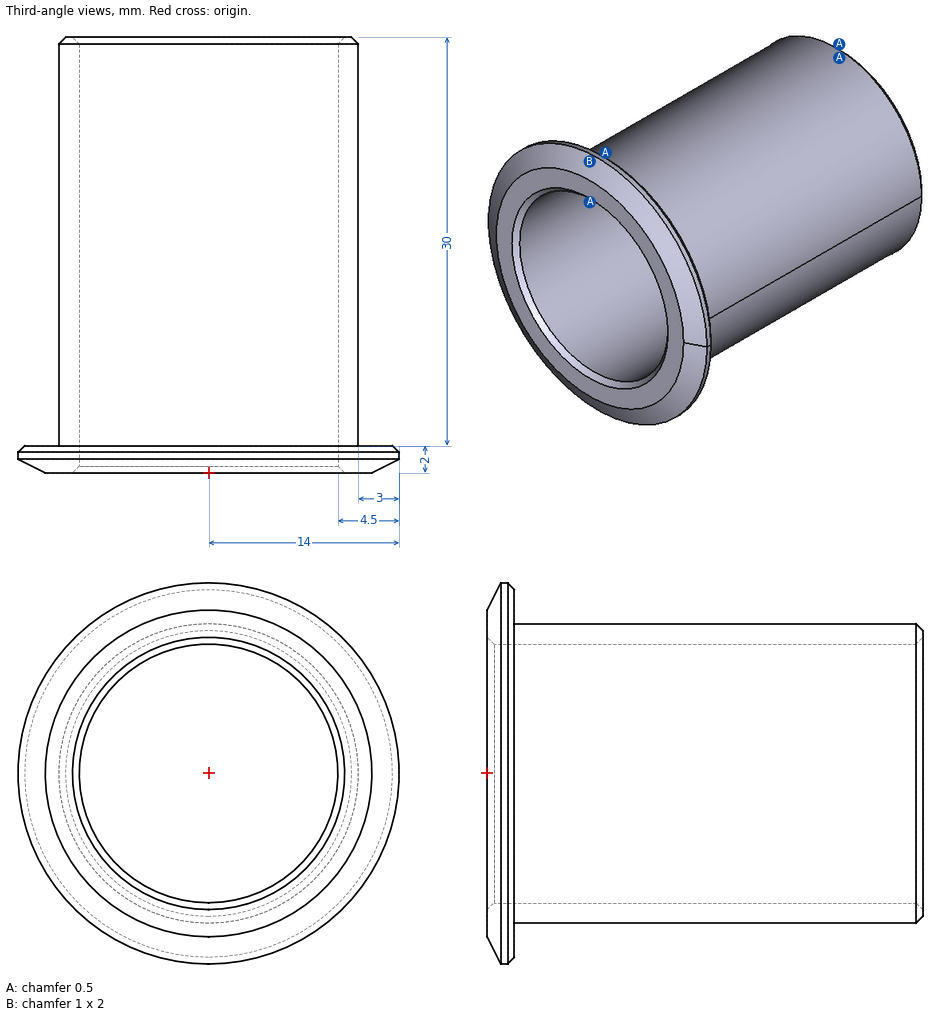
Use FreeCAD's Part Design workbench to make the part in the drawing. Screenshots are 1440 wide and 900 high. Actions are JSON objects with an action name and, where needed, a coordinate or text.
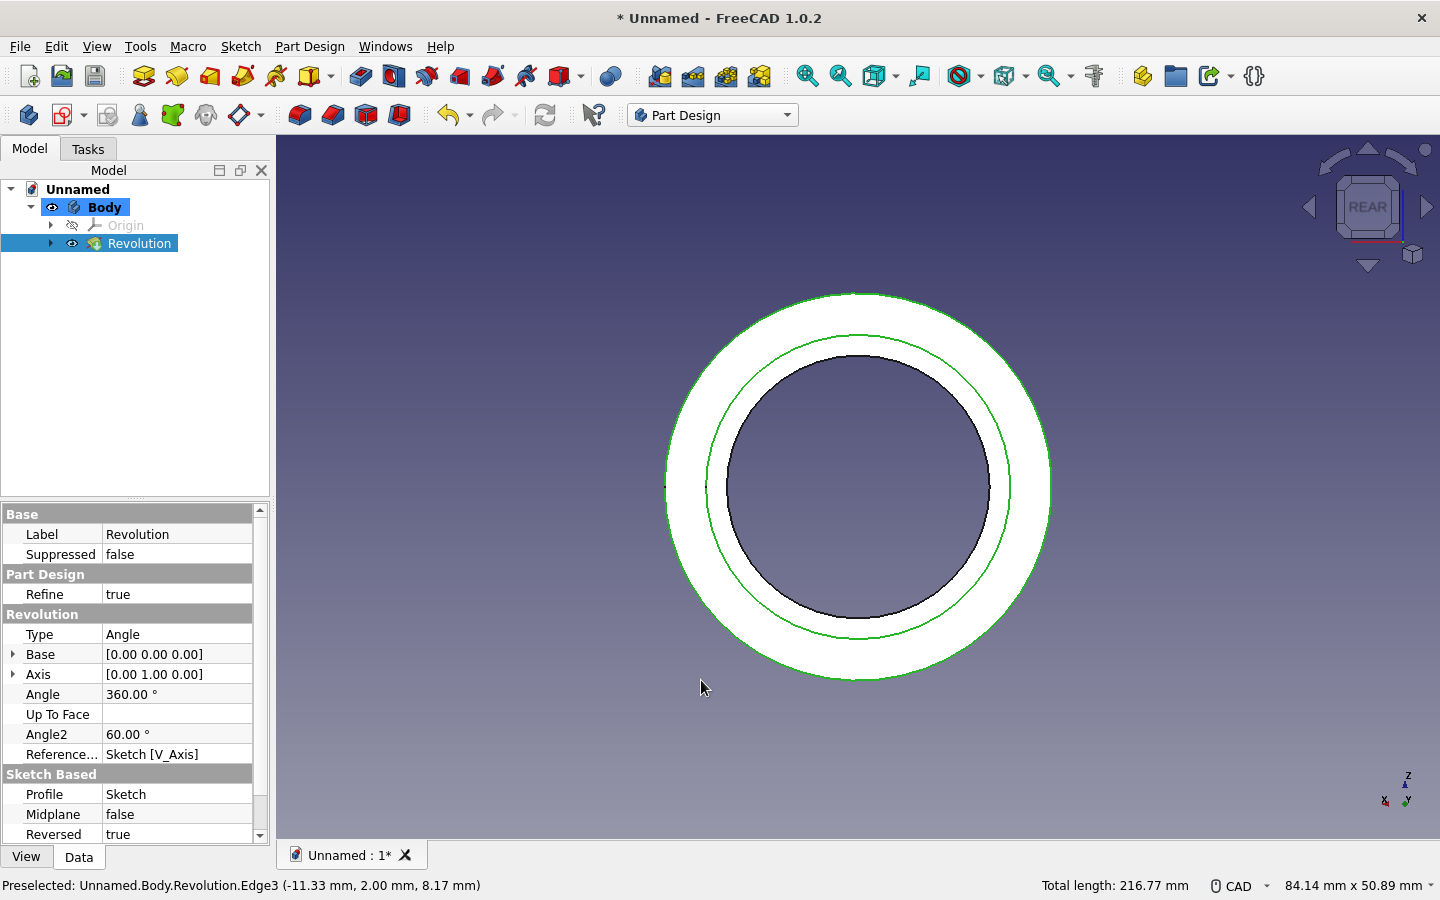
{"action": "left_click", "coordinate": [990, 486], "text": "ctrl"}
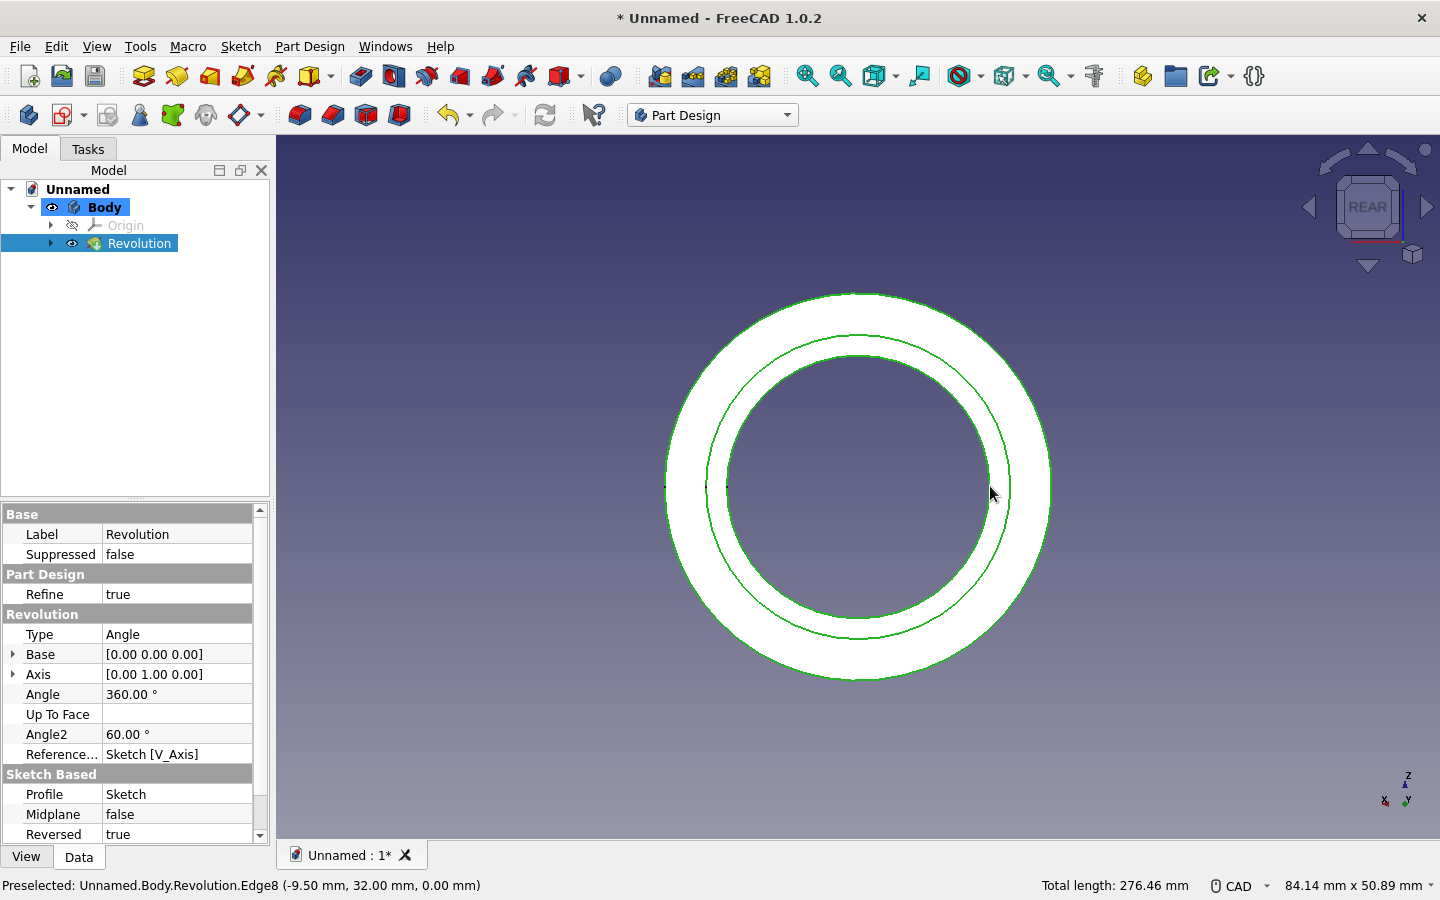
{"action": "left_click", "coordinate": [333, 116]}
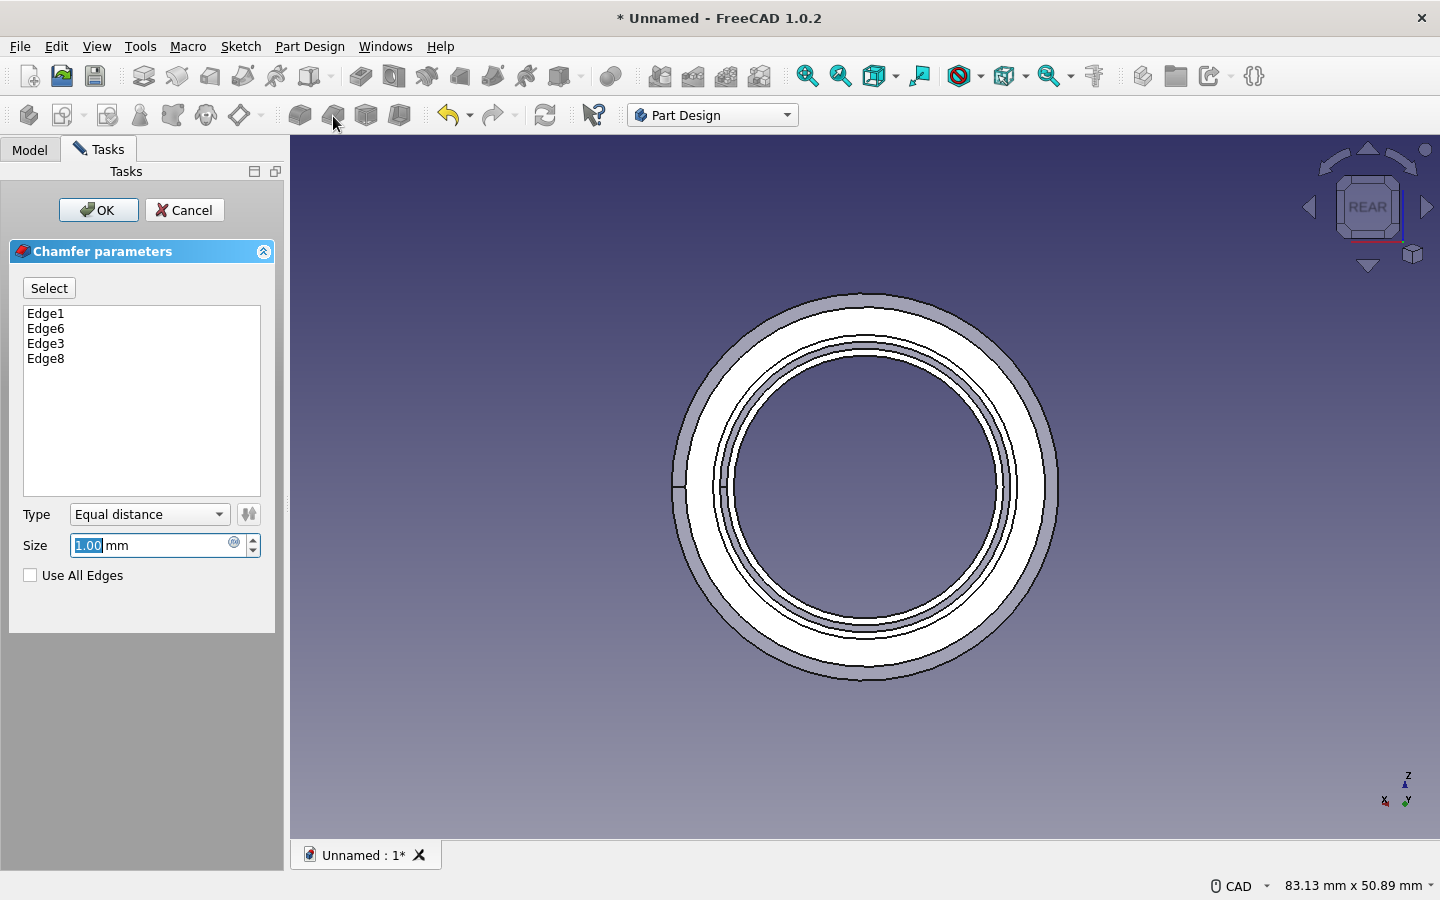
{"action": "type", "text": "0.5"}
{"action": "key", "text": "Tab"}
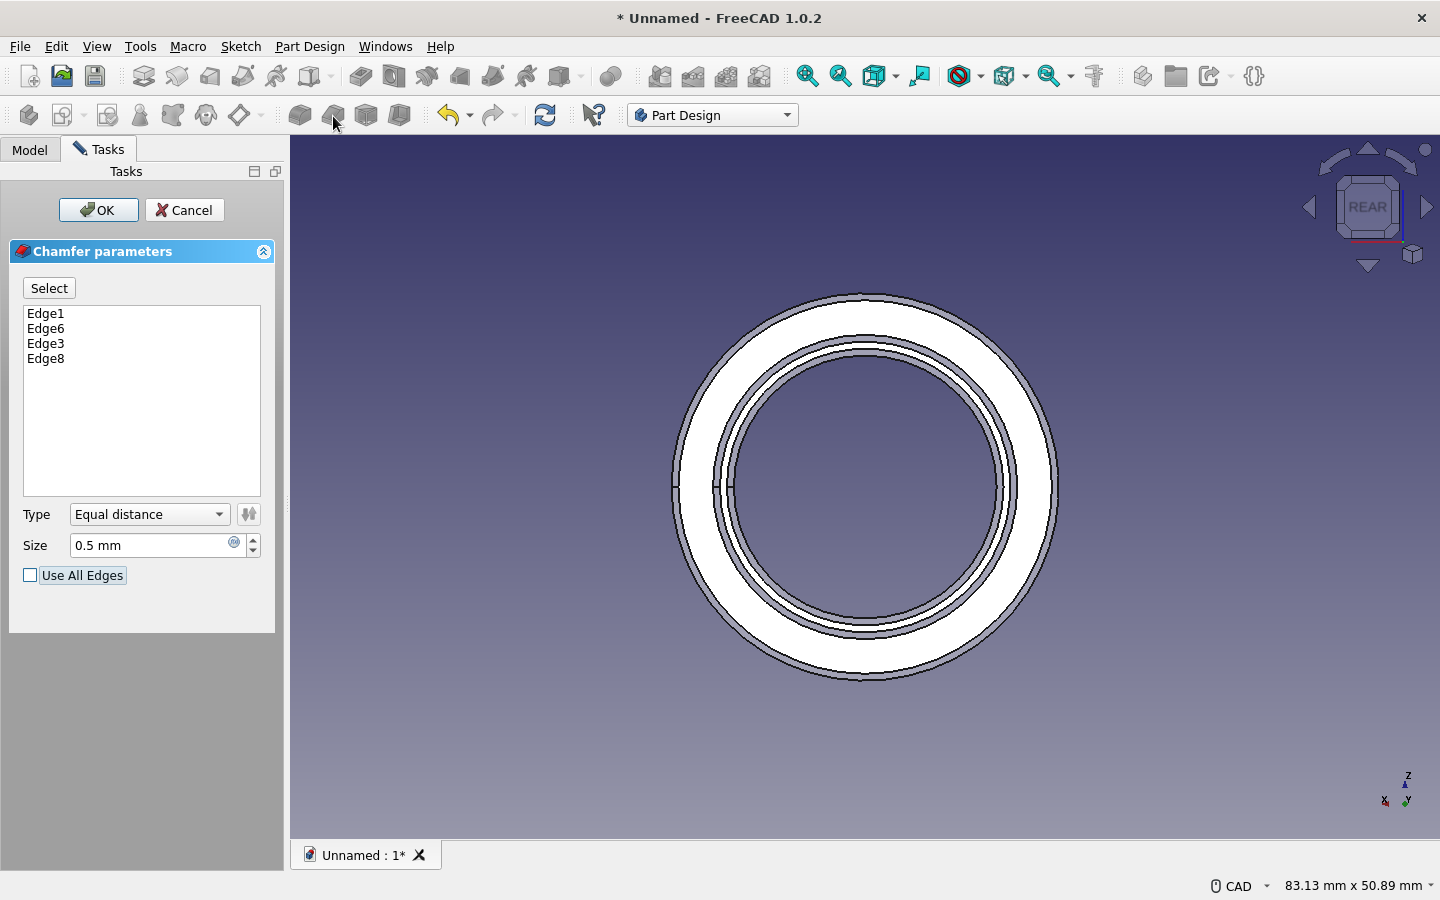
{"action": "left_click", "coordinate": [99, 210]}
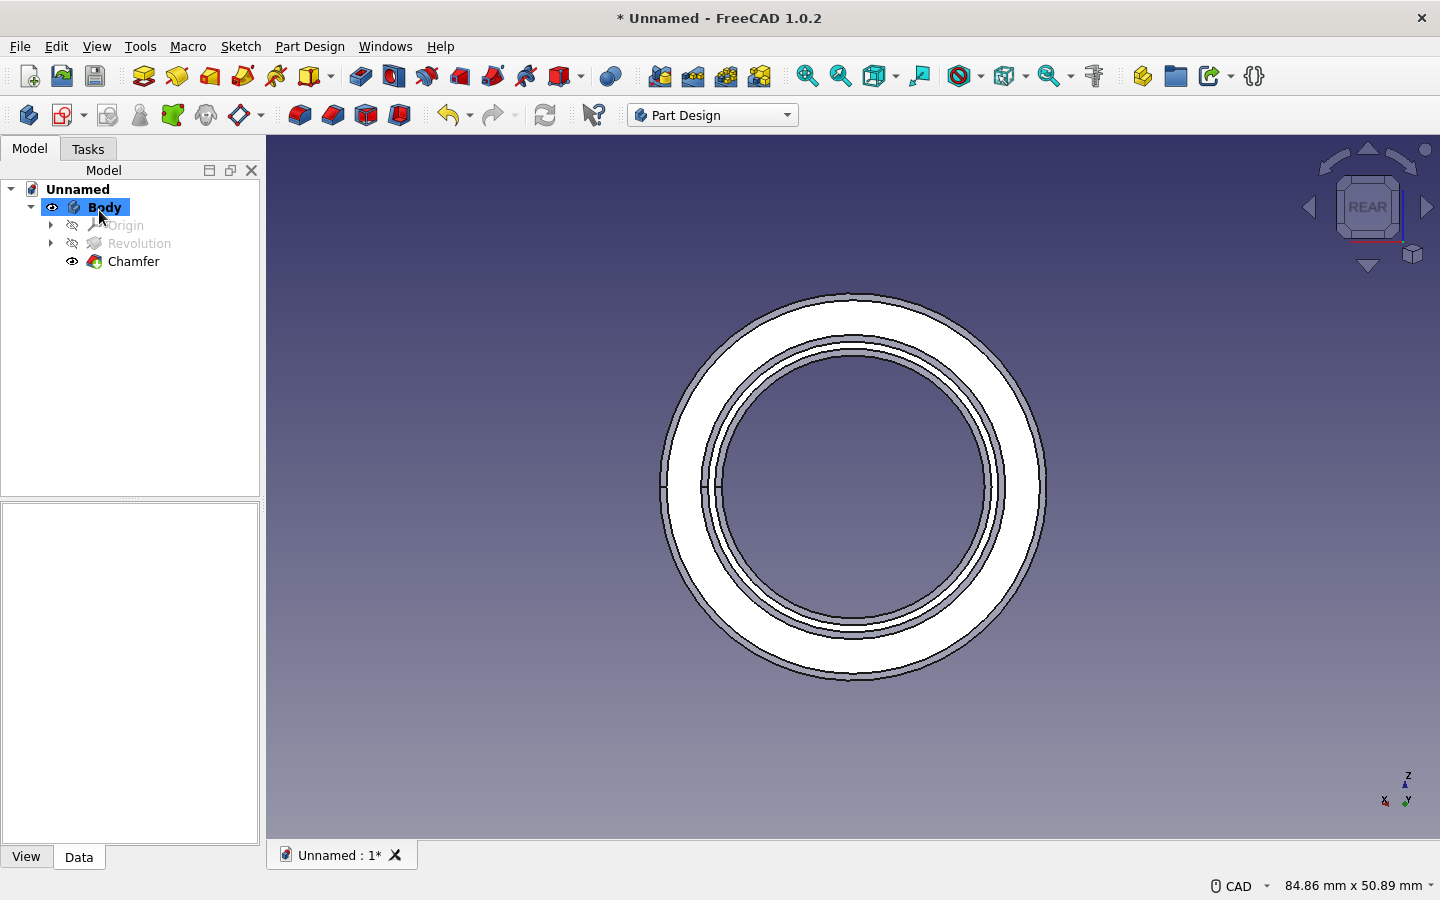
{"action": "key", "text": "0"}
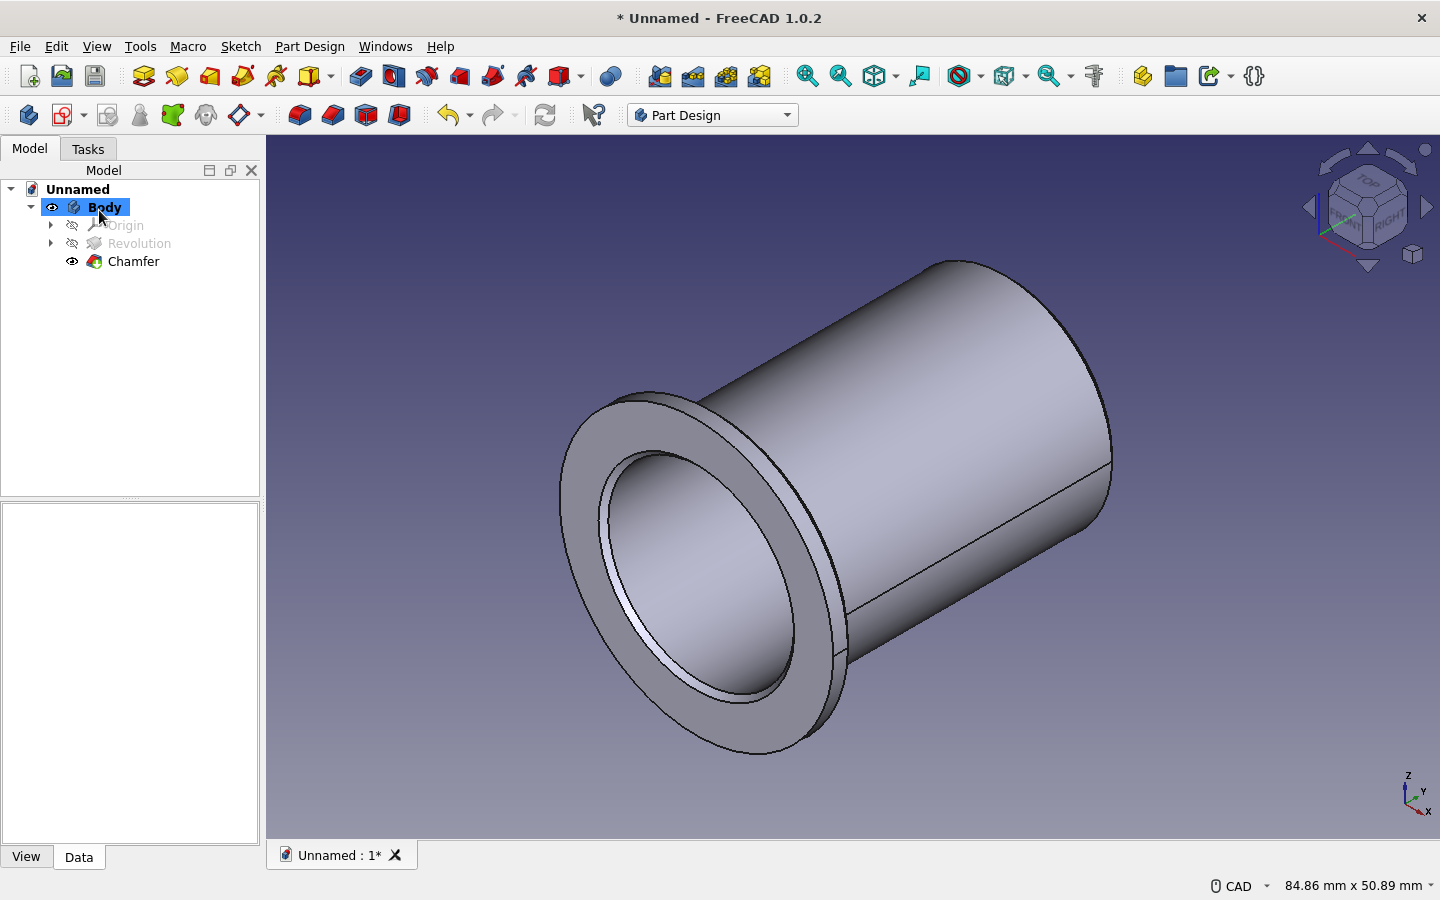
{"action": "left_click", "coordinate": [654, 401]}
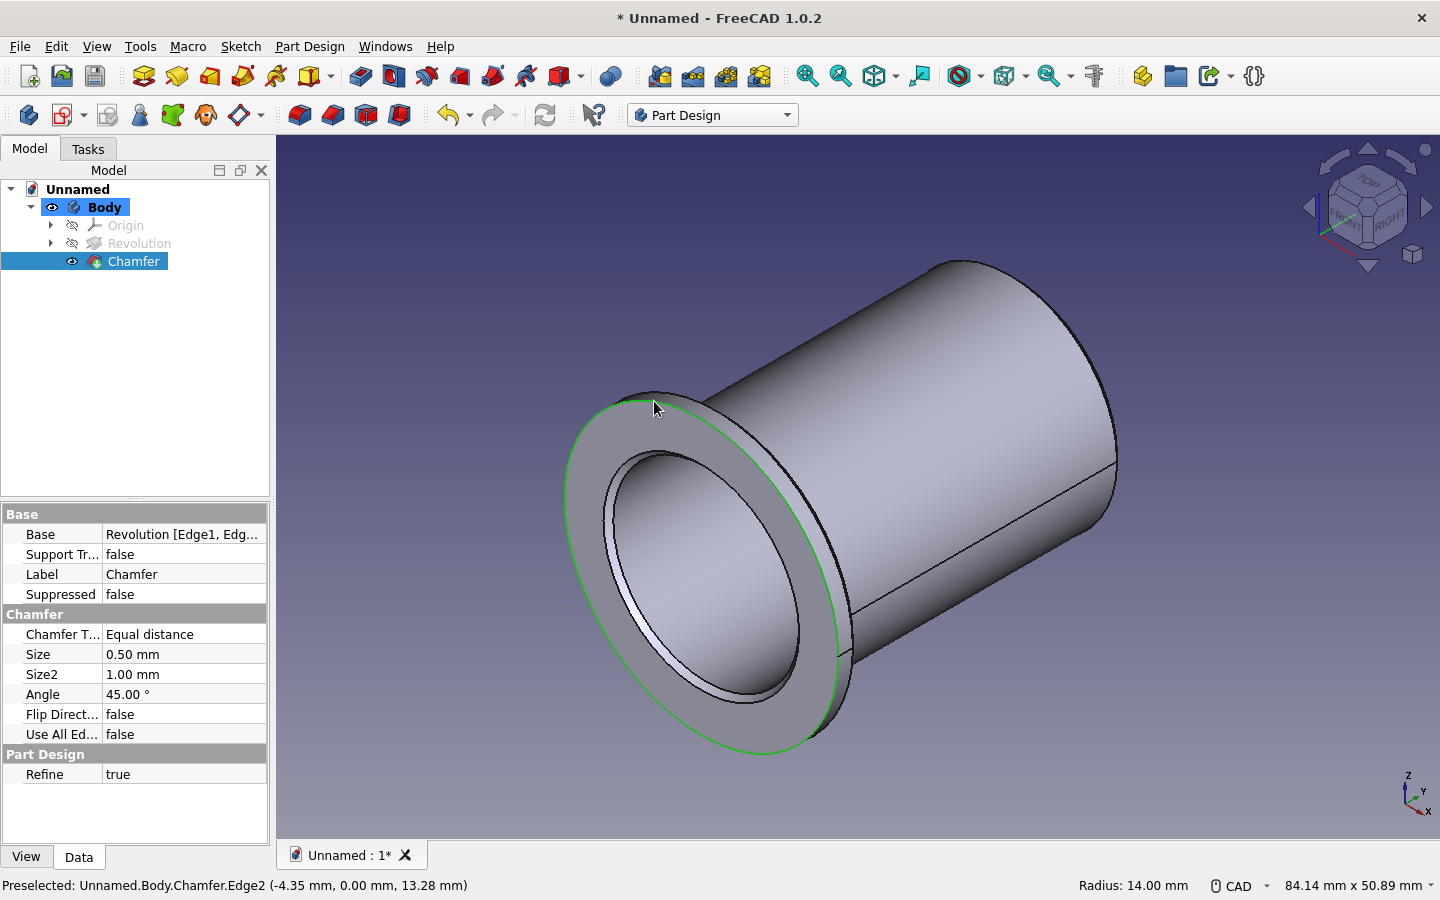
{"action": "left_click", "coordinate": [333, 116]}